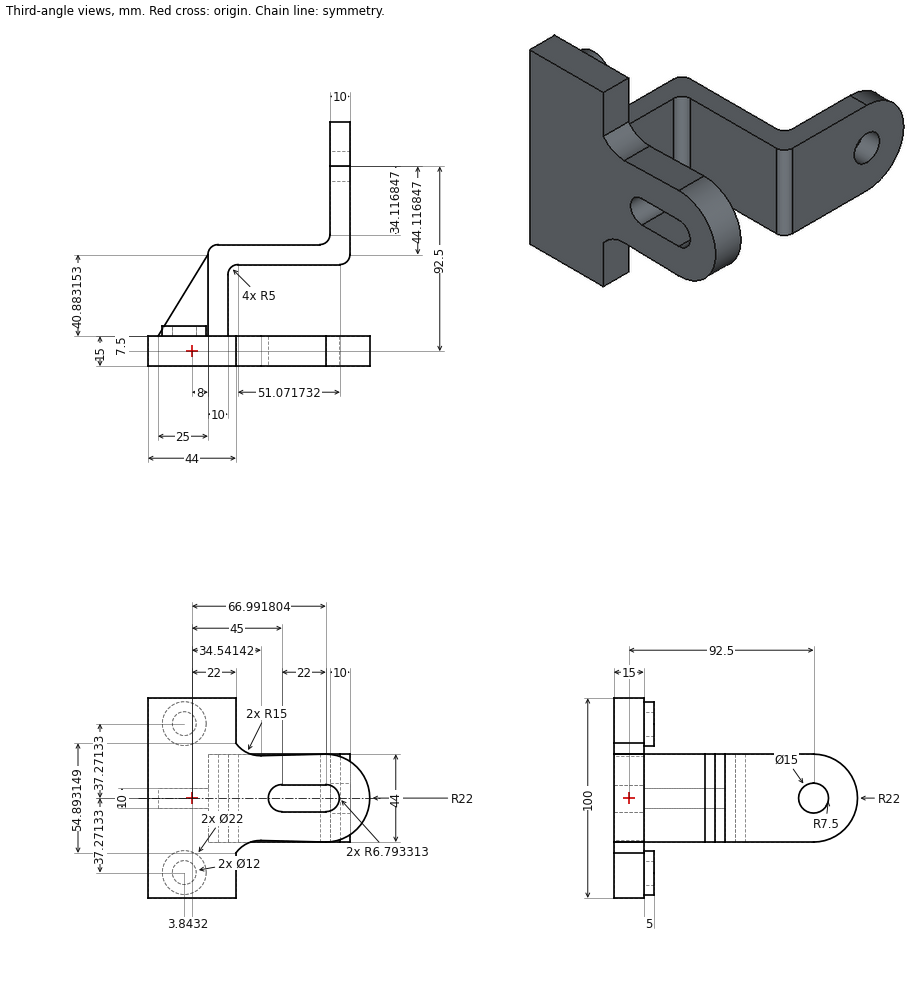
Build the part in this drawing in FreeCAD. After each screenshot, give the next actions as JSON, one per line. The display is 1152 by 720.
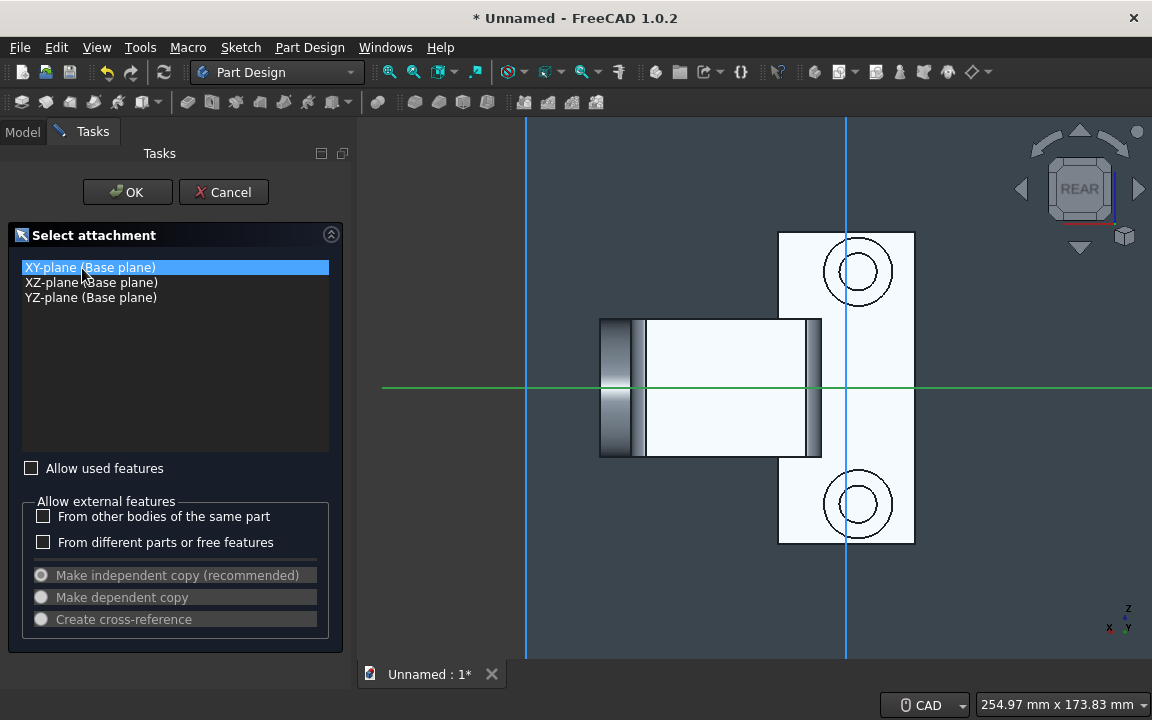
{"action": "left_click", "coordinate": [128, 192]}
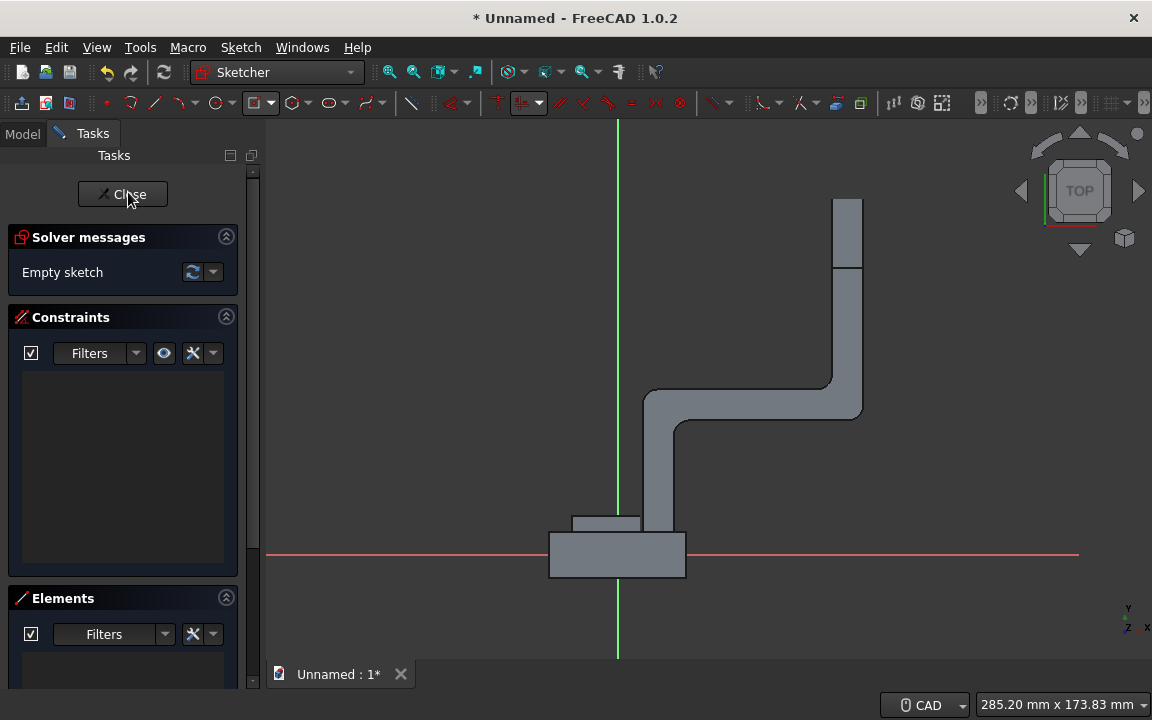
{"action": "left_click", "coordinate": [70, 104]}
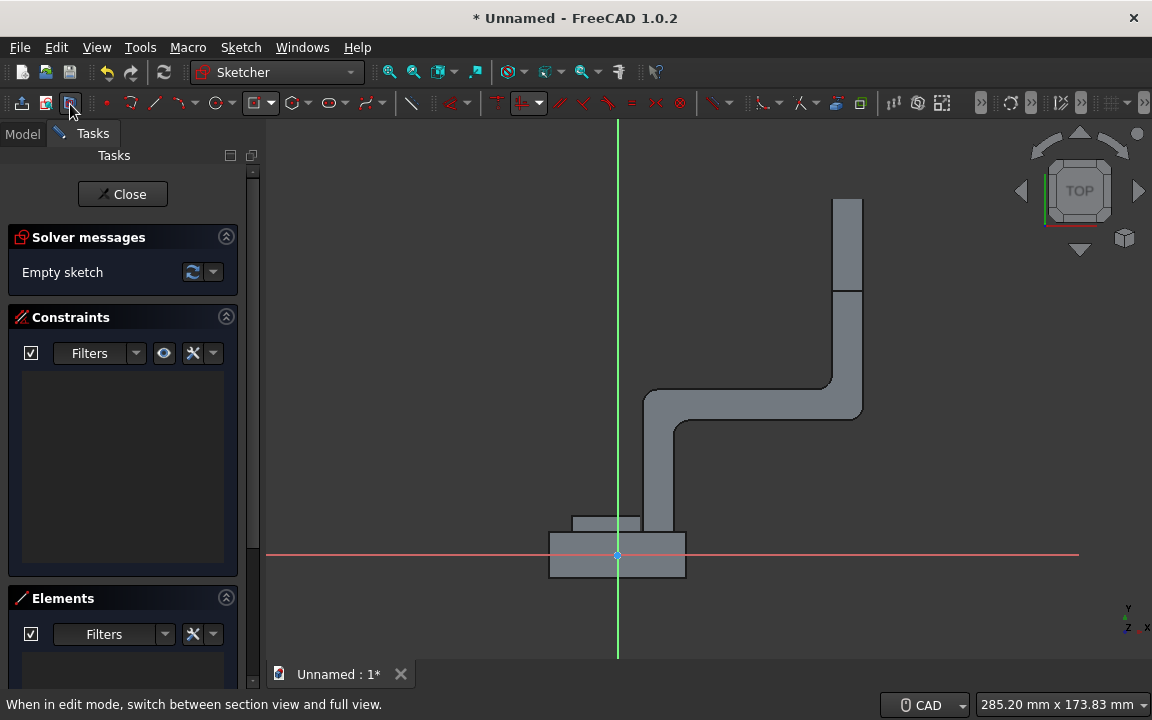
{"action": "scroll", "coordinate": [574, 554], "scroll_direction": "up", "scroll_amount": 4}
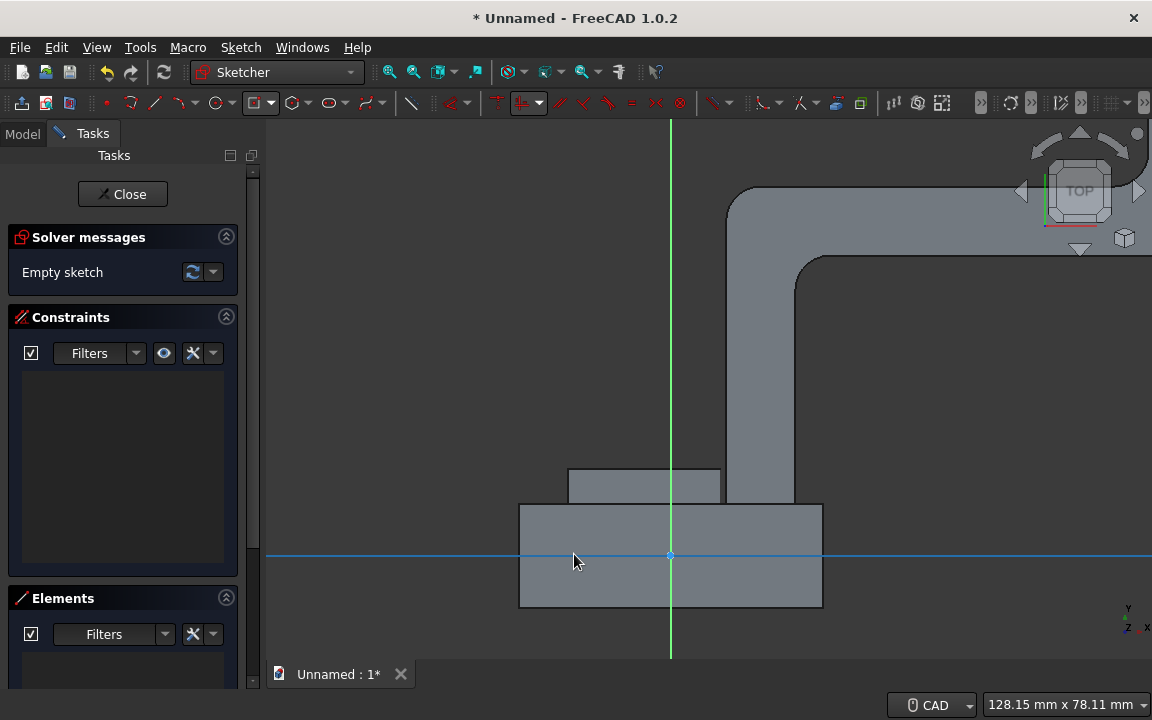
{"action": "left_click", "coordinate": [132, 104]}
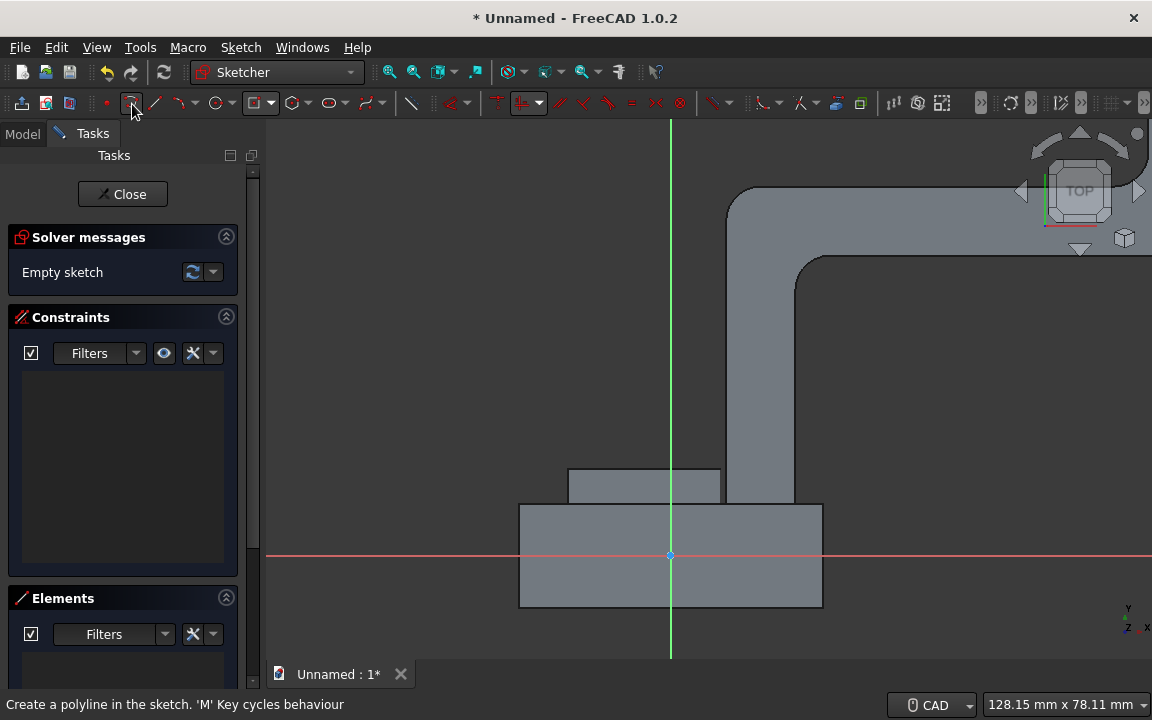
{"action": "left_click", "coordinate": [726, 504]}
{"action": "left_click", "coordinate": [726, 221]}
{"action": "left_click", "coordinate": [553, 504]}
{"action": "left_click", "coordinate": [726, 505]}
{"action": "key", "text": "Escape"}
{"action": "key", "text": "Escape"}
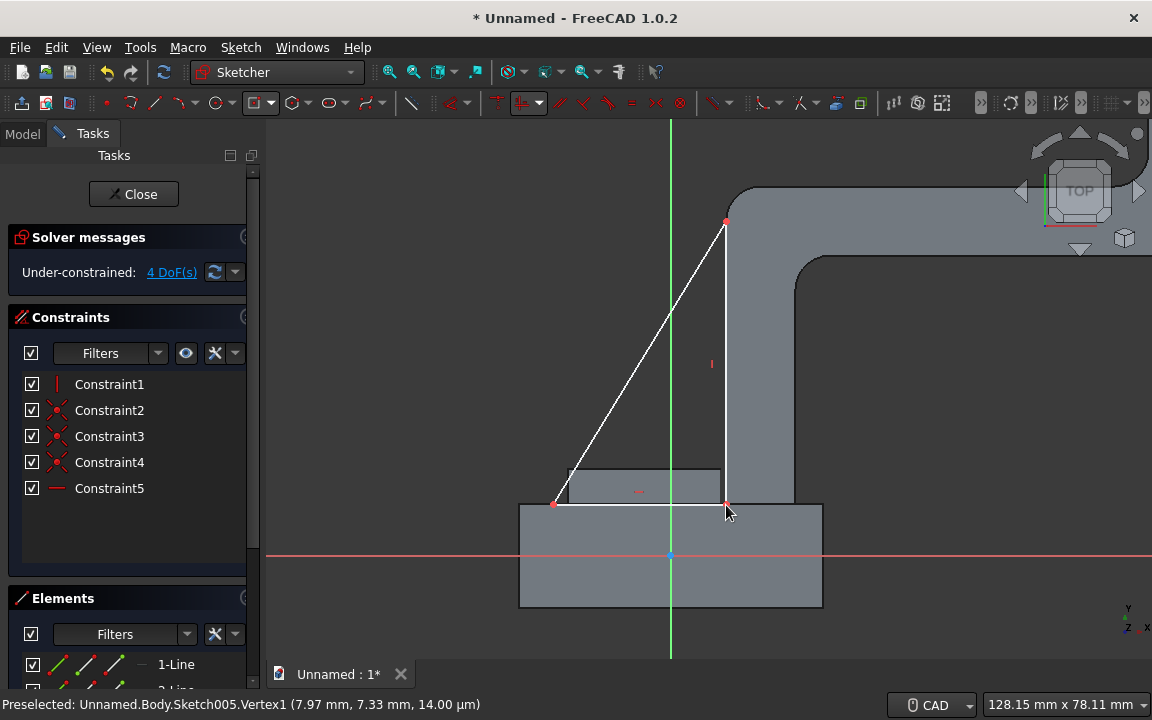
{"action": "left_click", "coordinate": [450, 104]}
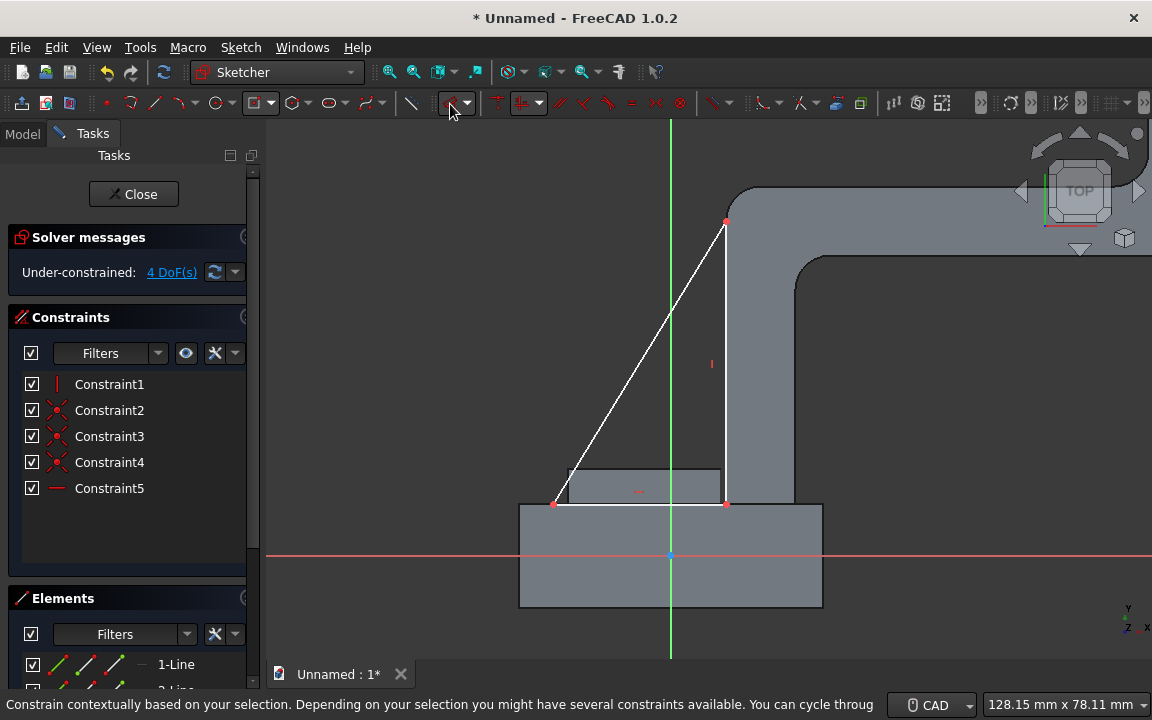
{"action": "left_click", "coordinate": [605, 505]}
{"action": "left_click", "coordinate": [639, 539]}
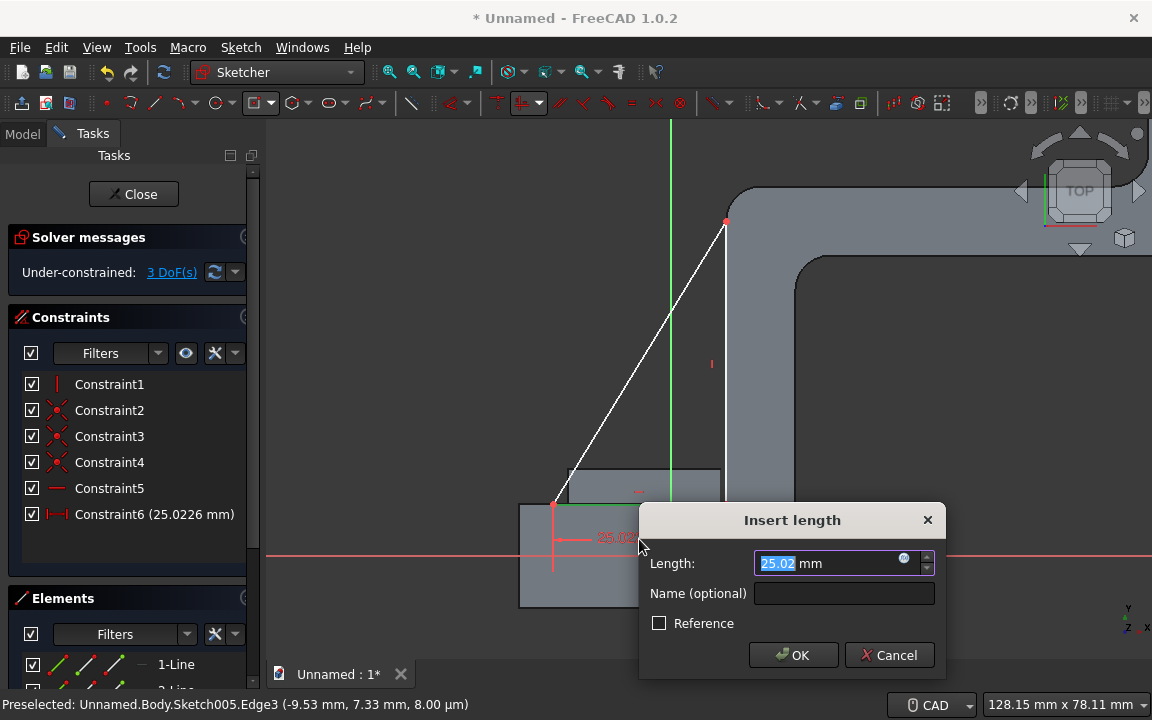
{"action": "type", "text": "25"}
{"action": "key", "text": "Return"}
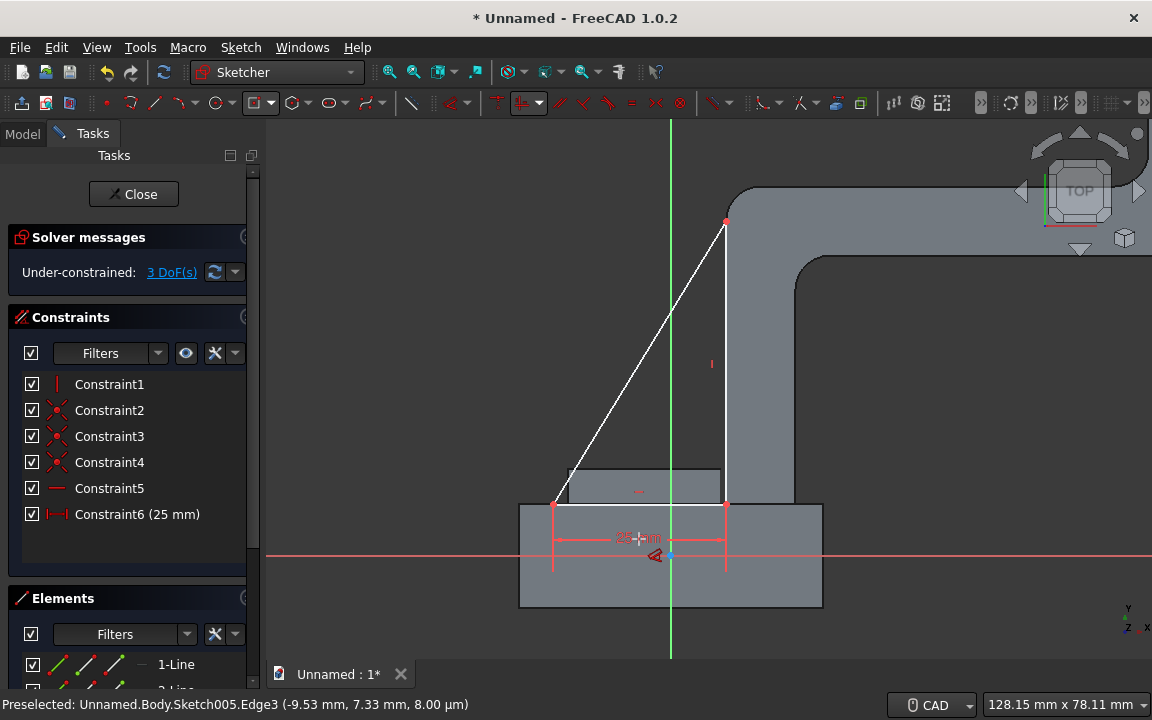
{"action": "left_click", "coordinate": [726, 505]}
{"action": "left_click", "coordinate": [698, 590]}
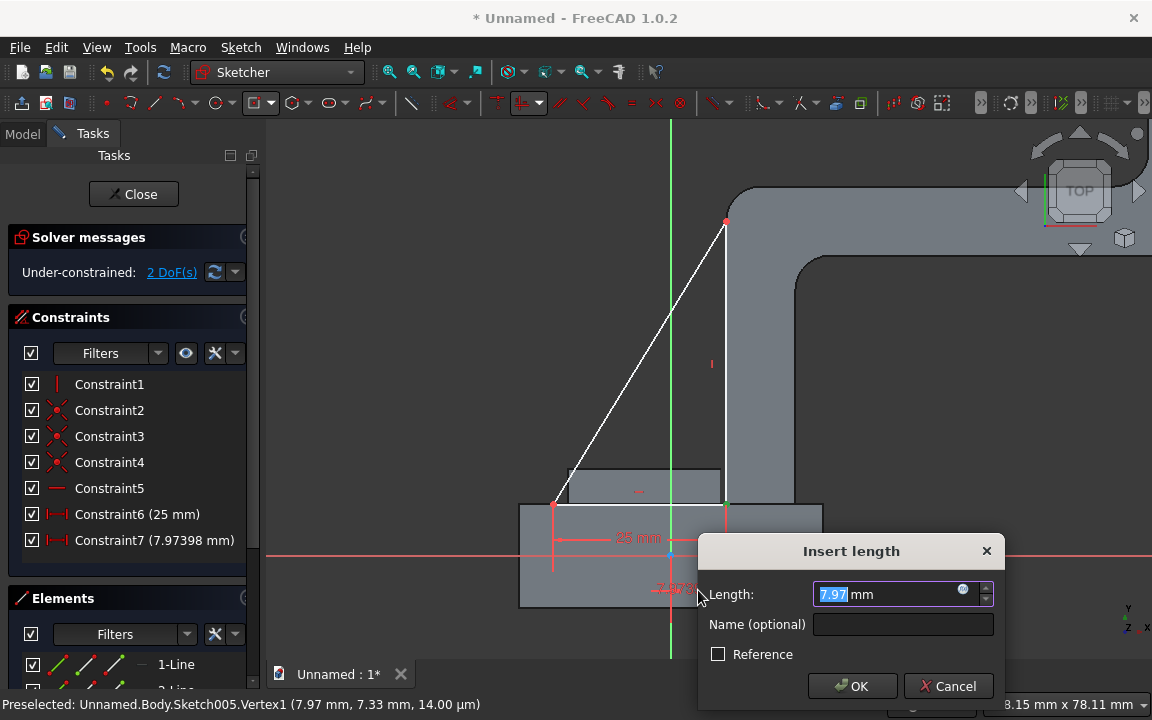
{"action": "type", "text": "8"}
{"action": "key", "text": "Return"}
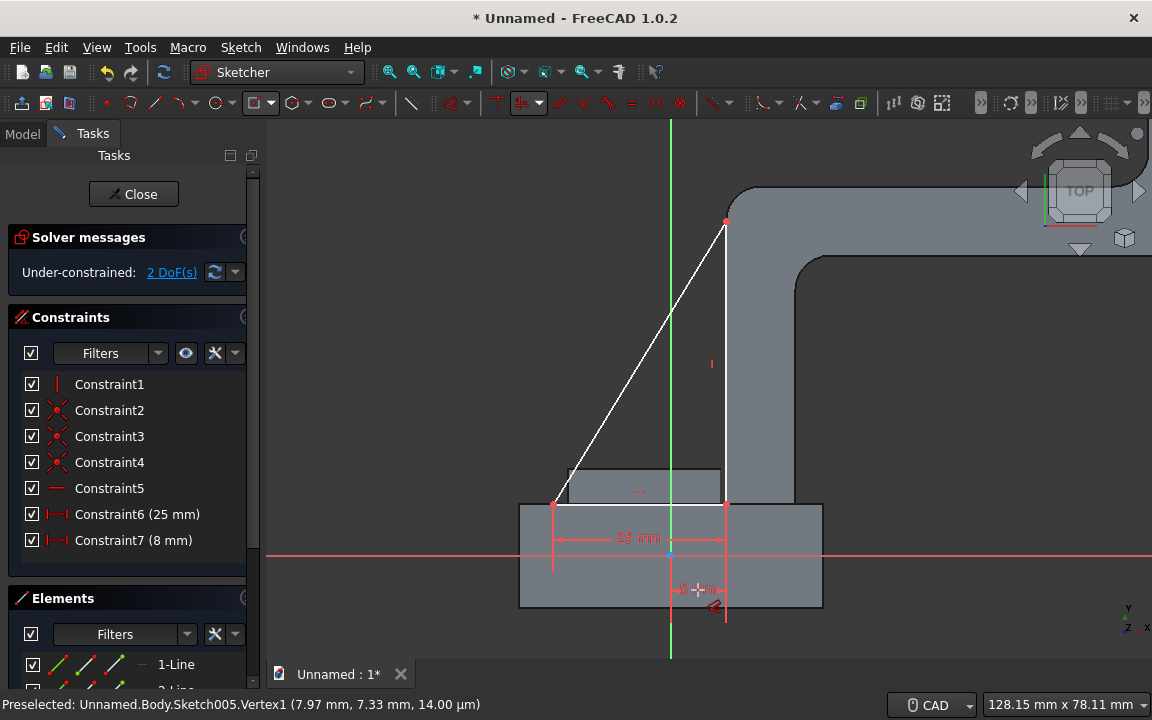
{"action": "left_click", "coordinate": [726, 505]}
{"action": "left_click", "coordinate": [760, 530]}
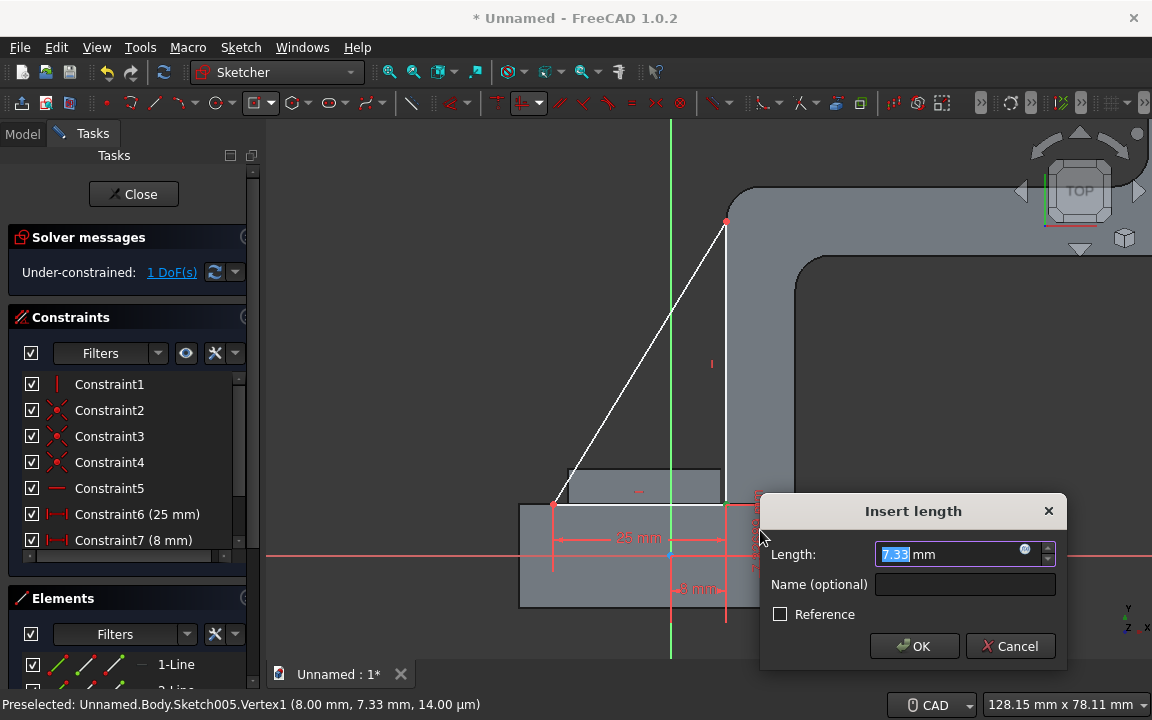
{"action": "type", "text": "7.5"}
{"action": "key", "text": "Return"}